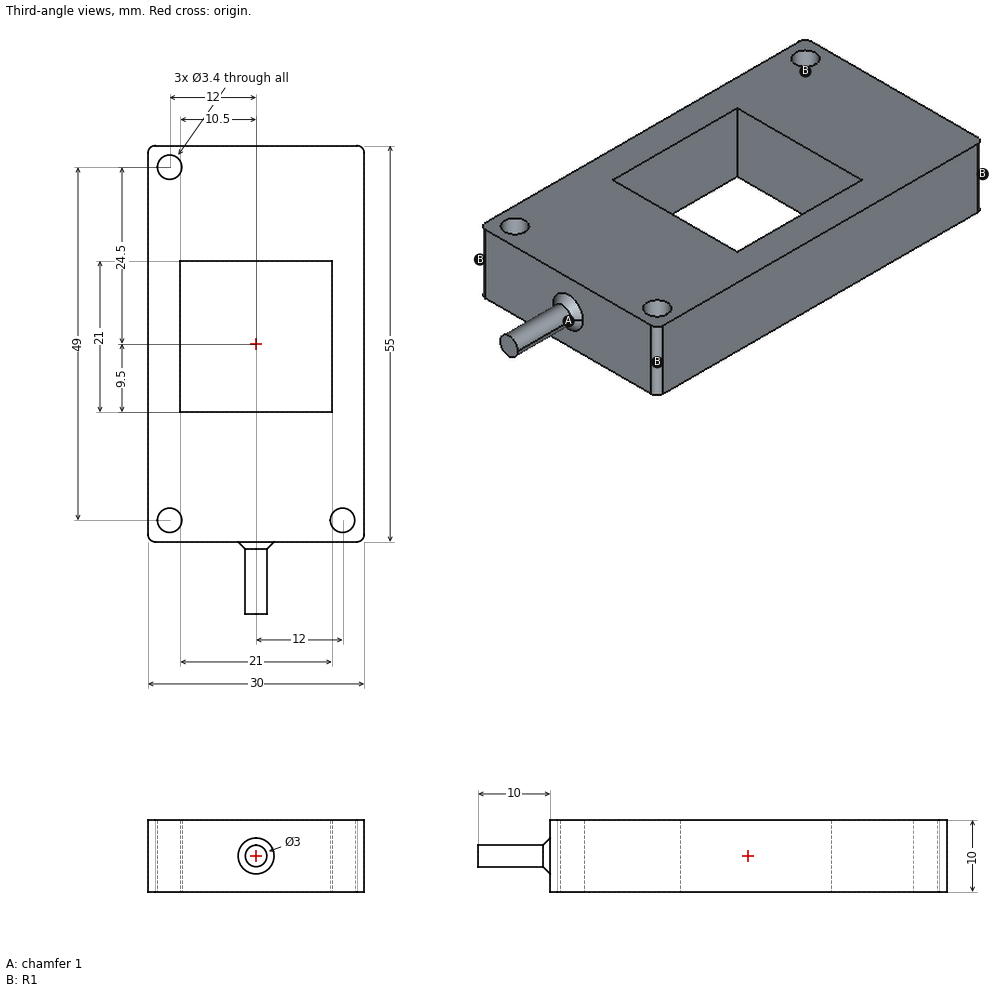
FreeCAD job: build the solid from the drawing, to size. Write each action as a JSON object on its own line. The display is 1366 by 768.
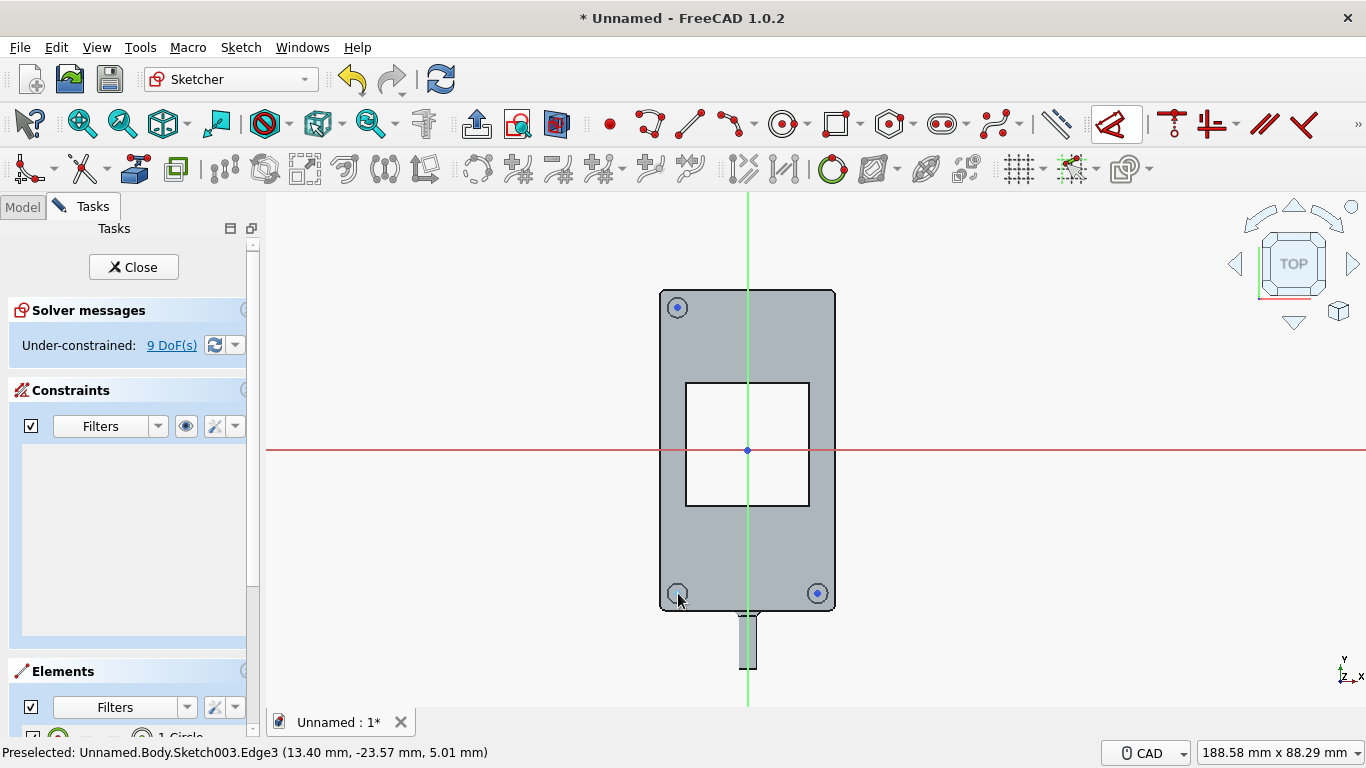
{"action": "scroll", "coordinate": [684, 301], "scroll_direction": "up", "scroll_amount": 2}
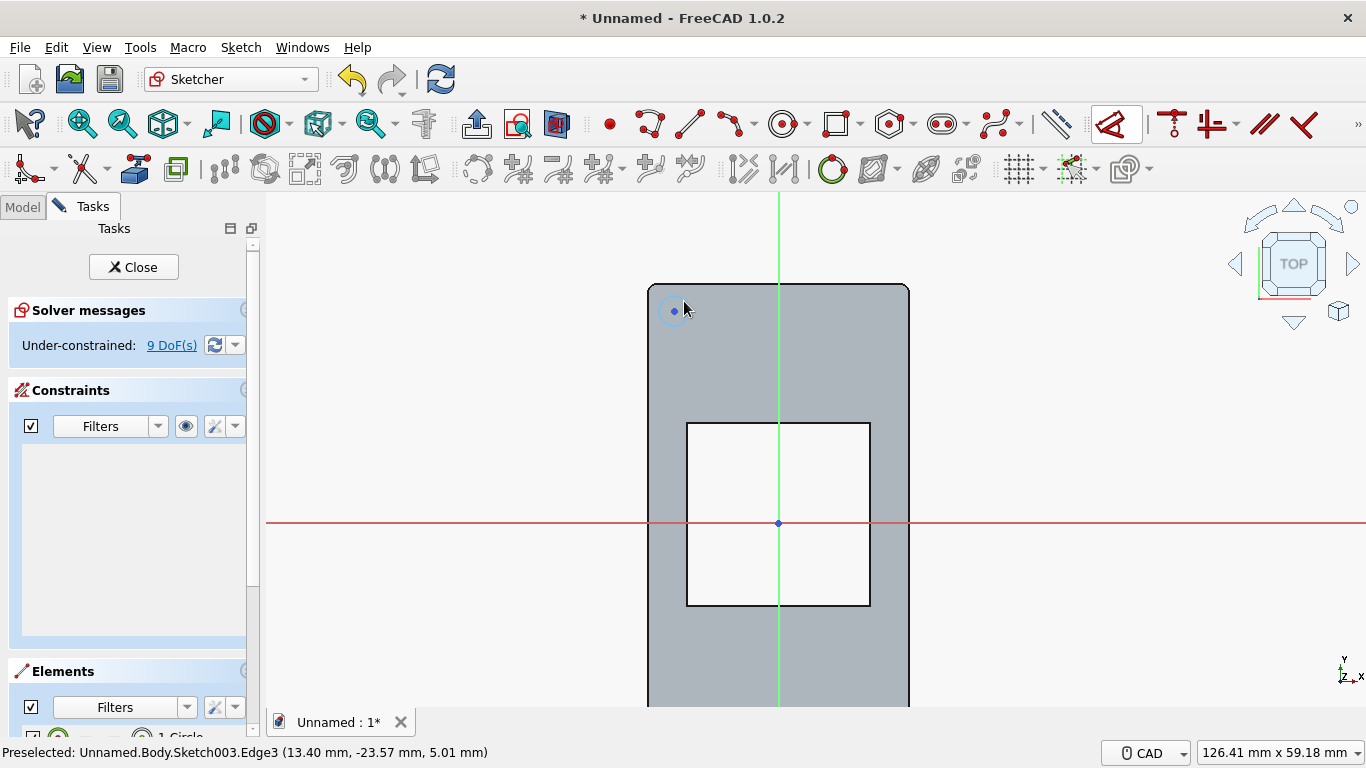
{"action": "left_click", "coordinate": [685, 301]}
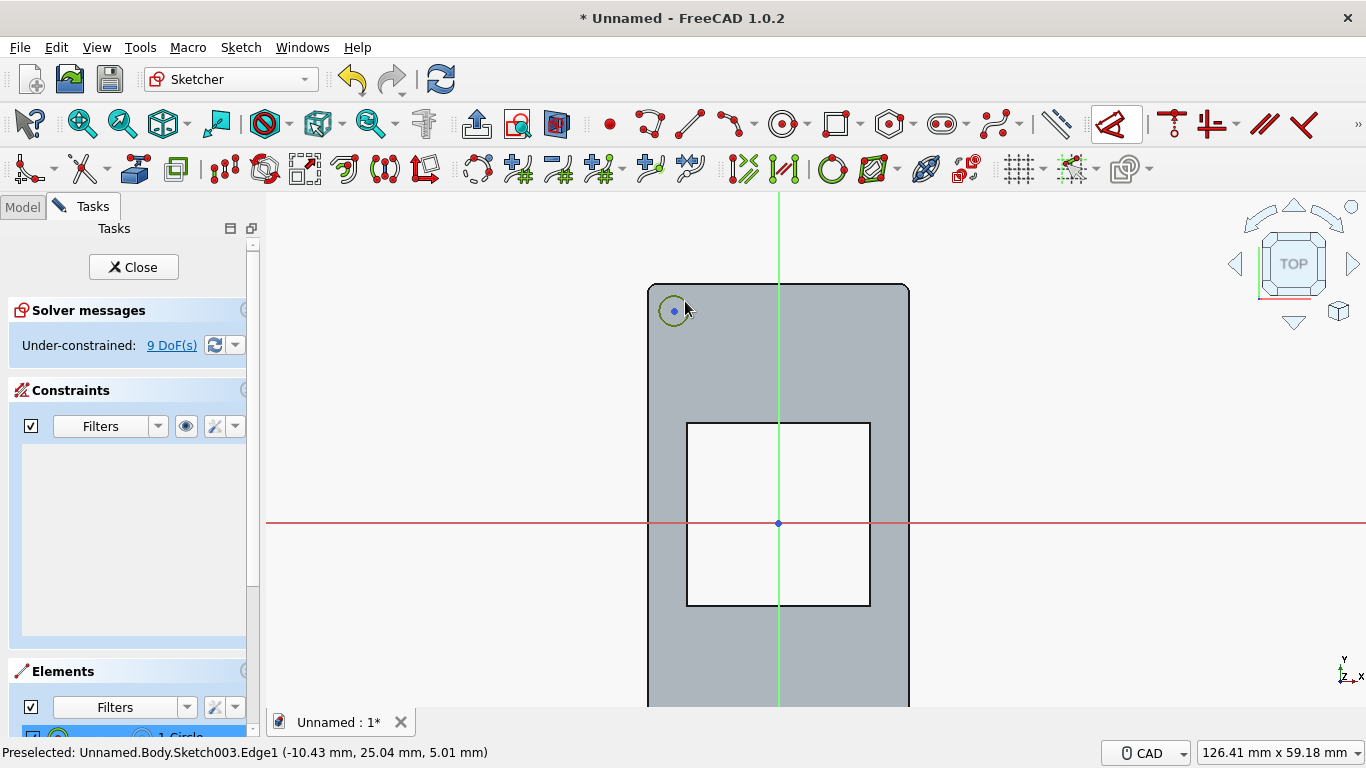
{"action": "scroll", "coordinate": [684, 299], "scroll_direction": "down", "scroll_amount": 2}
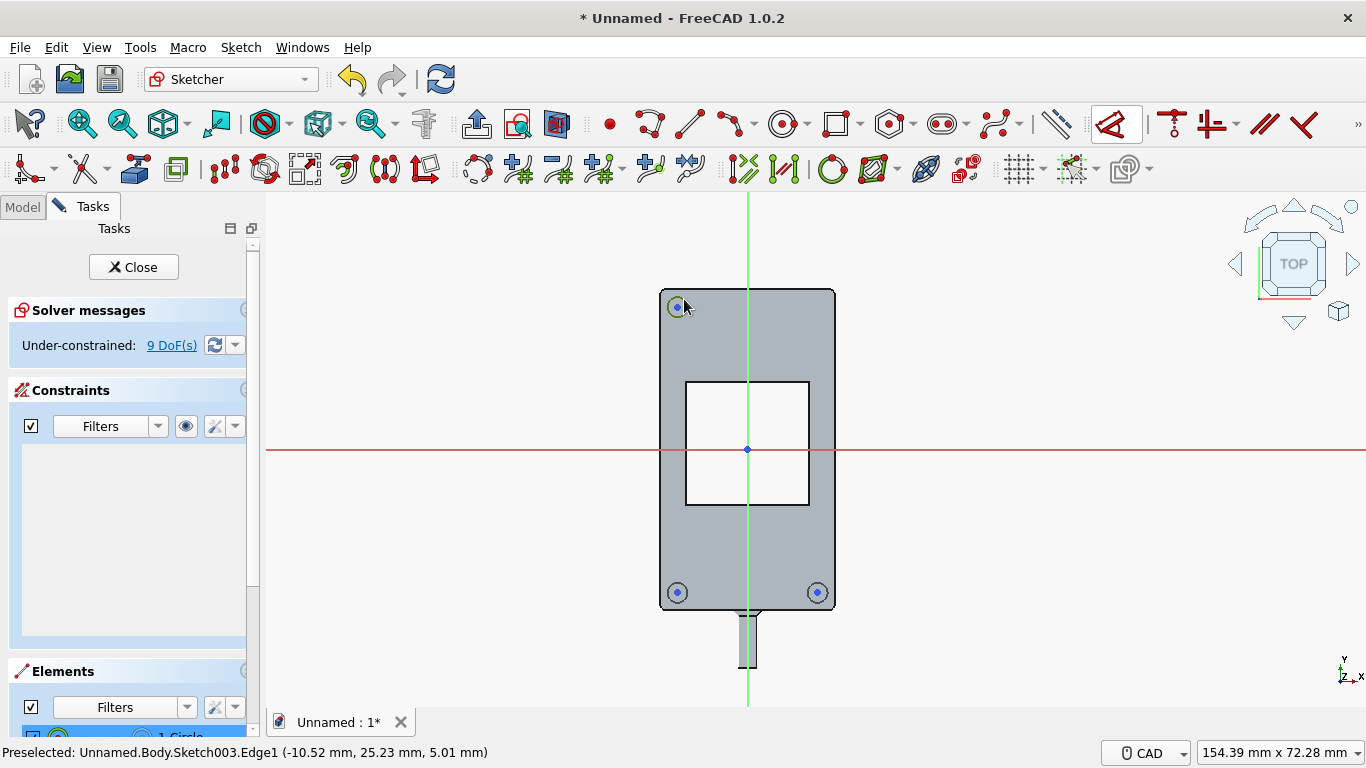
{"action": "scroll", "coordinate": [684, 586], "scroll_direction": "up", "scroll_amount": 2}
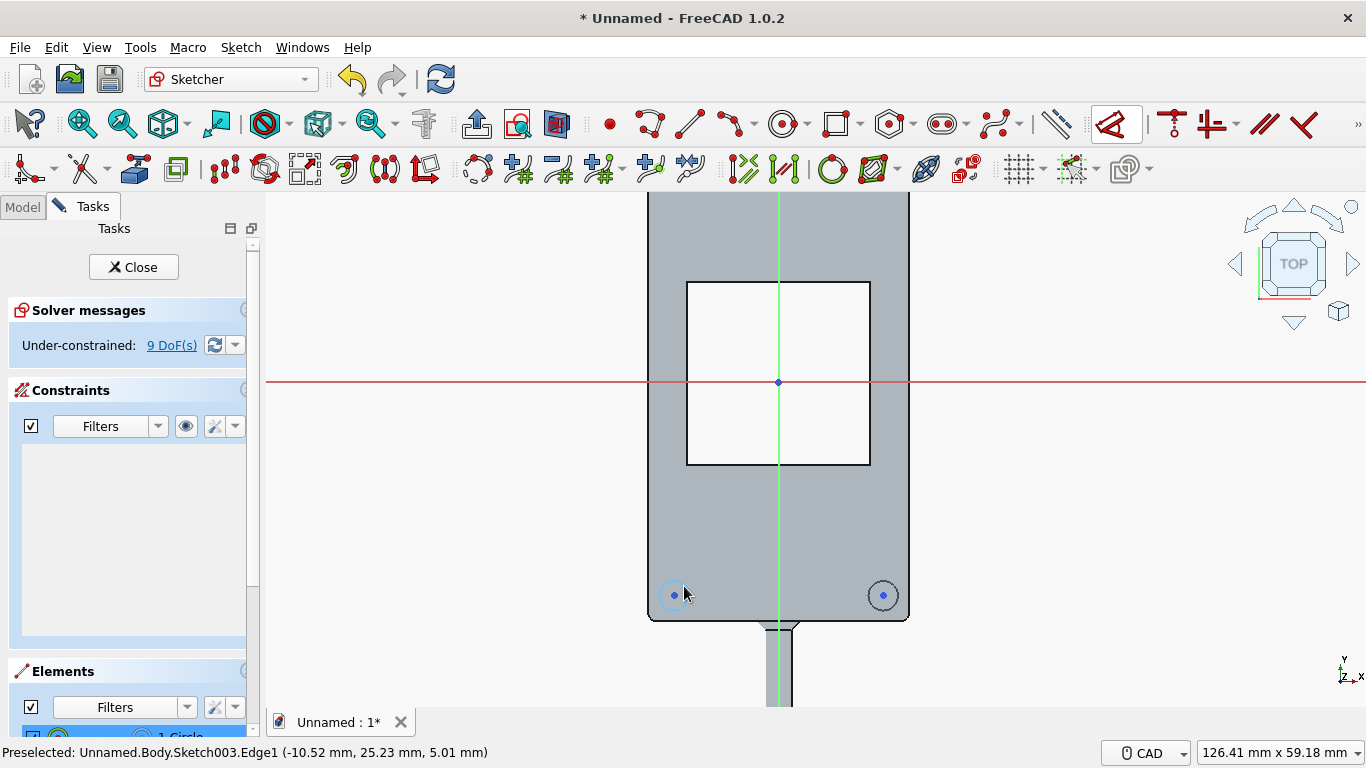
{"action": "left_click", "coordinate": [685, 585]}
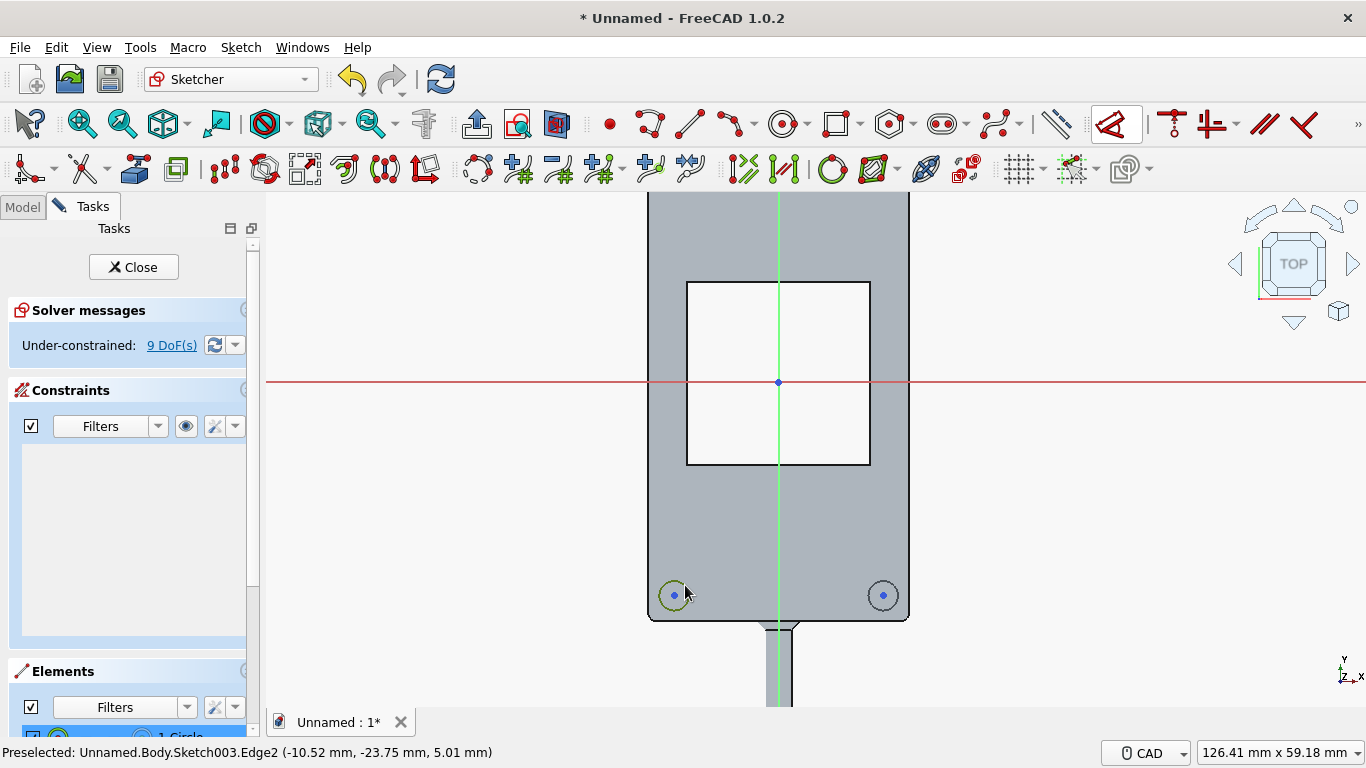
{"action": "left_click", "coordinate": [894, 585]}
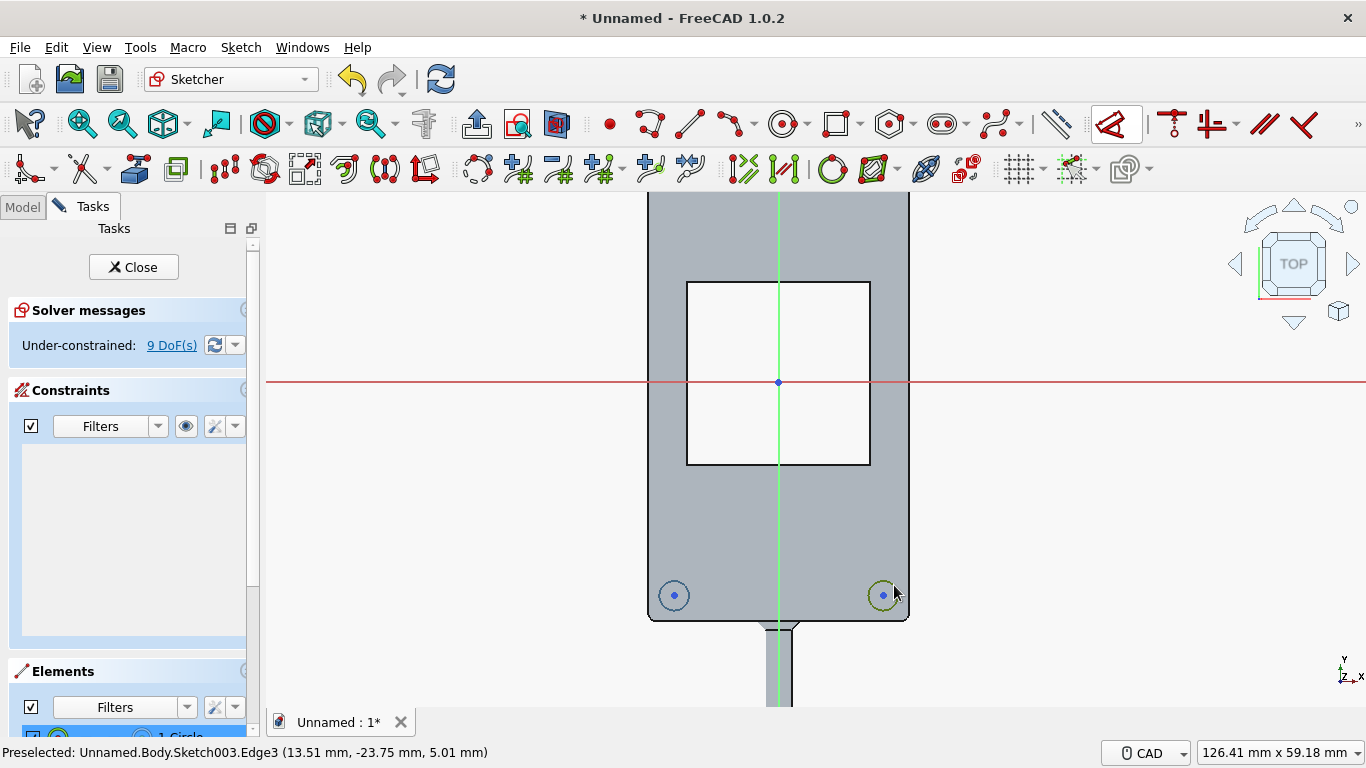
{"action": "key", "text": "e"}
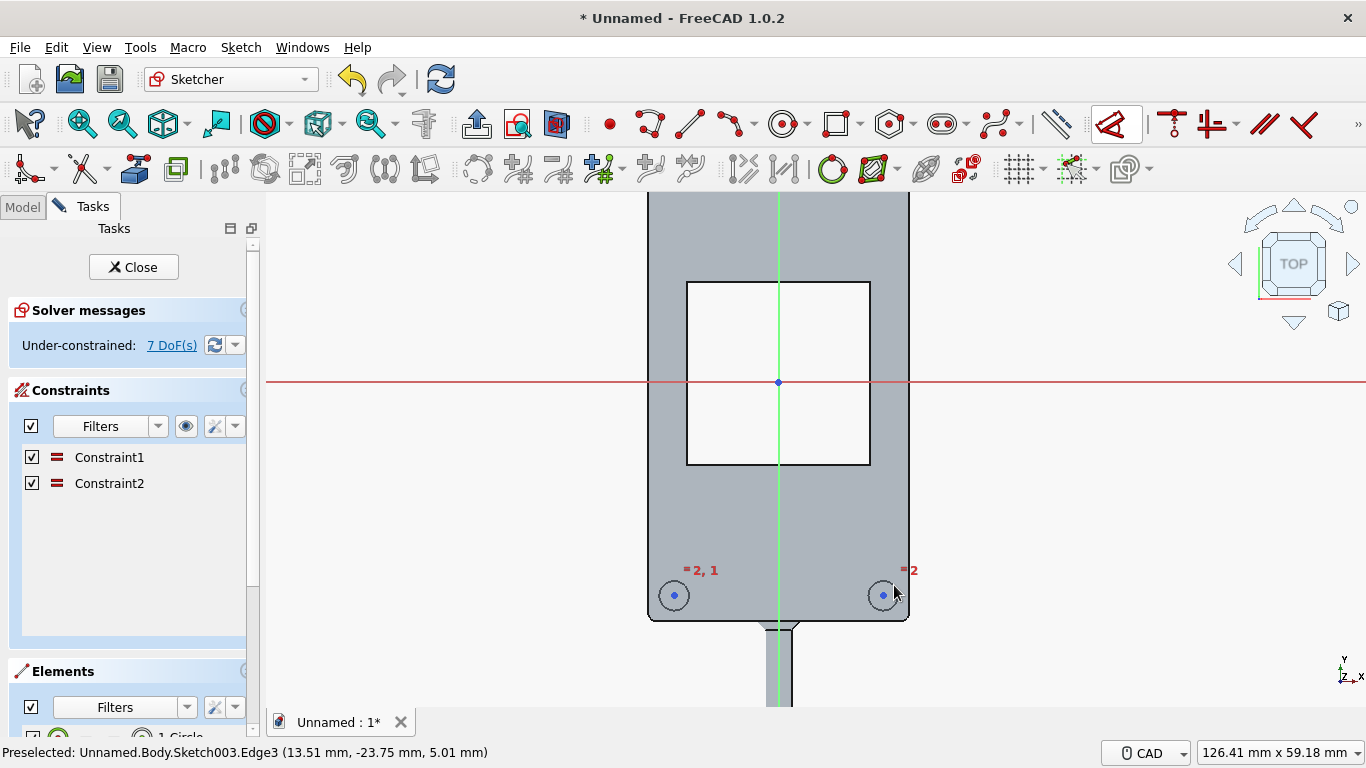
{"action": "scroll", "coordinate": [684, 587], "scroll_direction": "down", "scroll_amount": 2}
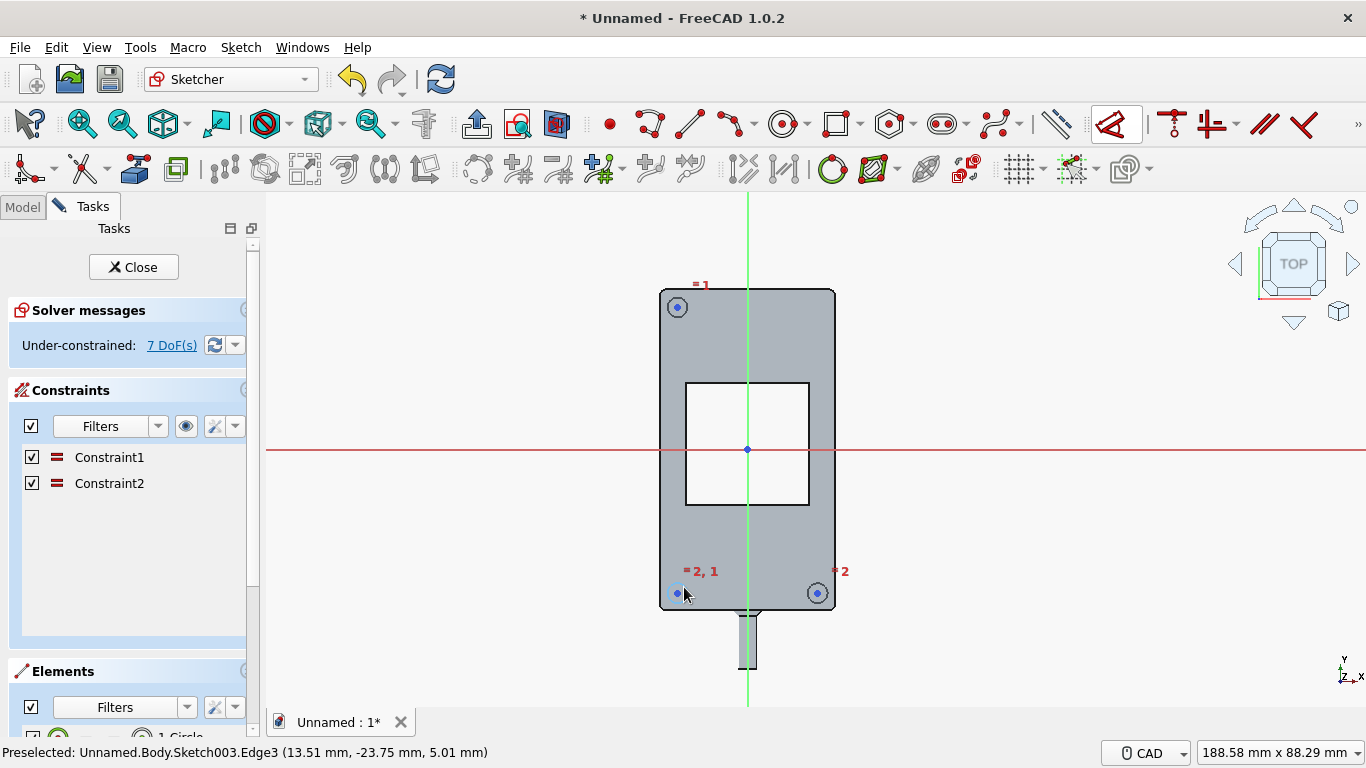
{"action": "left_click", "coordinate": [678, 307]}